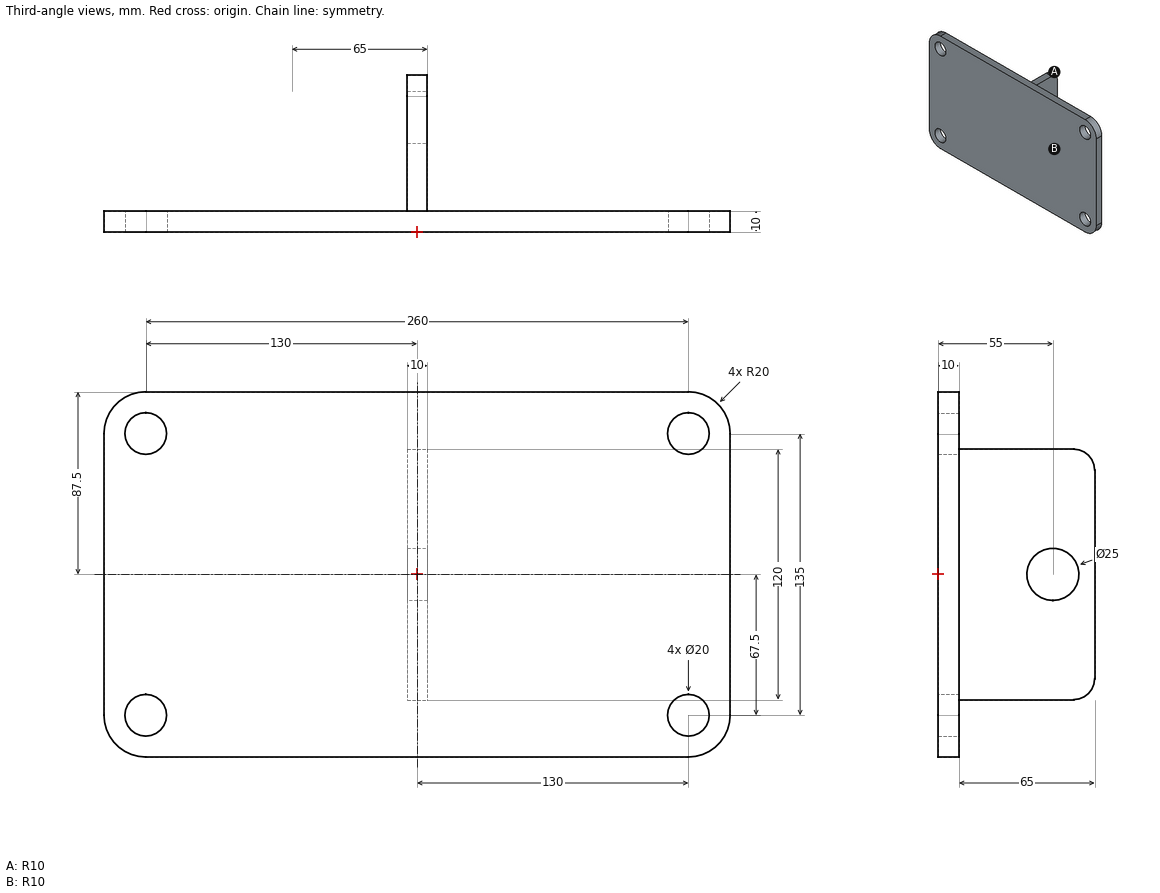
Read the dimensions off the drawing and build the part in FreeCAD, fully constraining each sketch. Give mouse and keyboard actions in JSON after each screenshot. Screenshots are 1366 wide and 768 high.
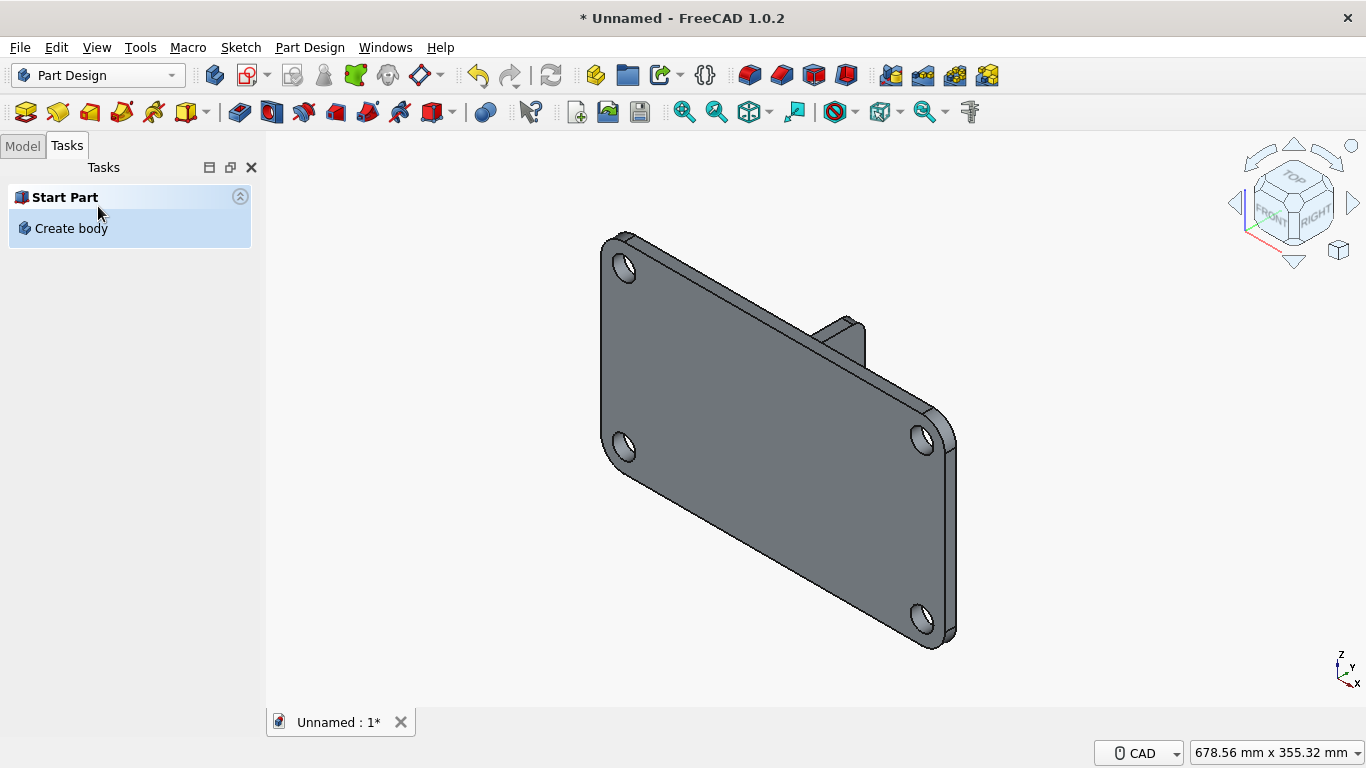
{"action": "key", "text": "3"}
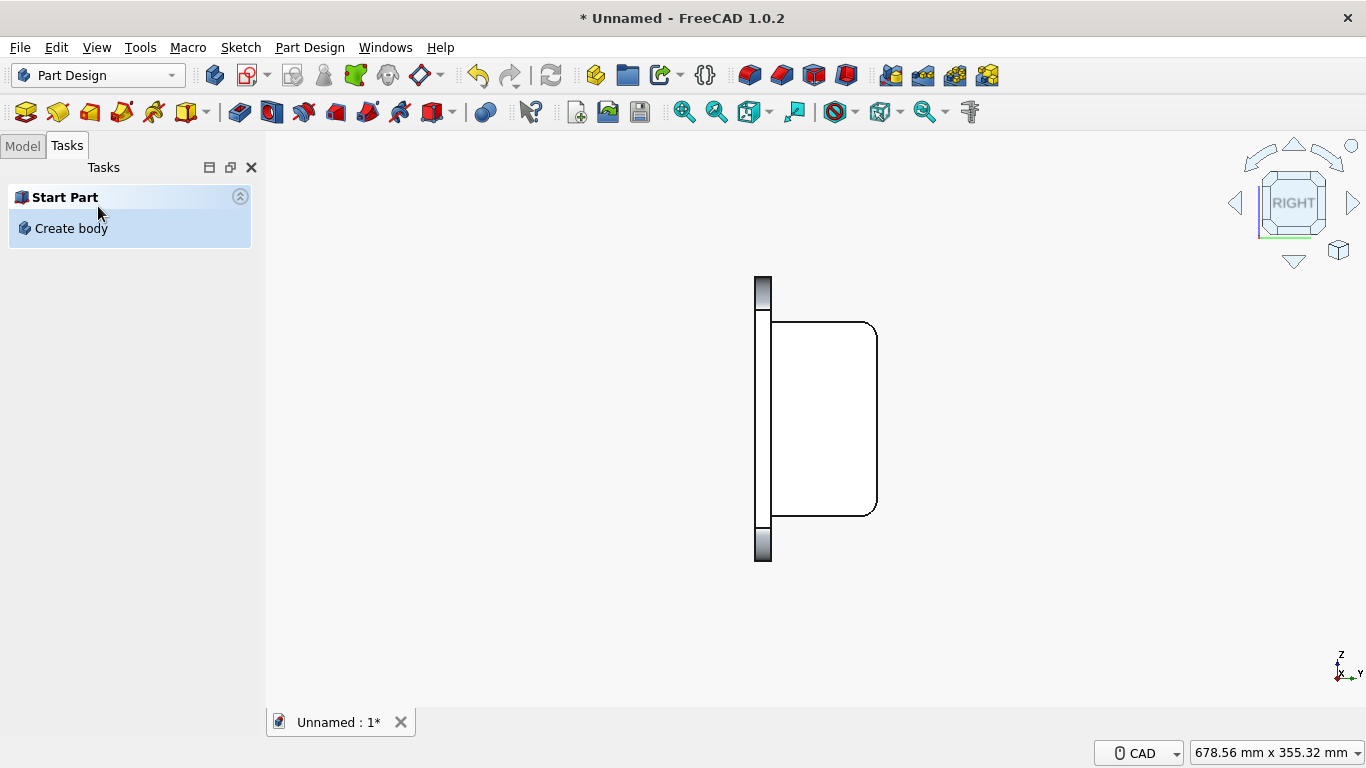
{"action": "left_click", "coordinate": [824, 446]}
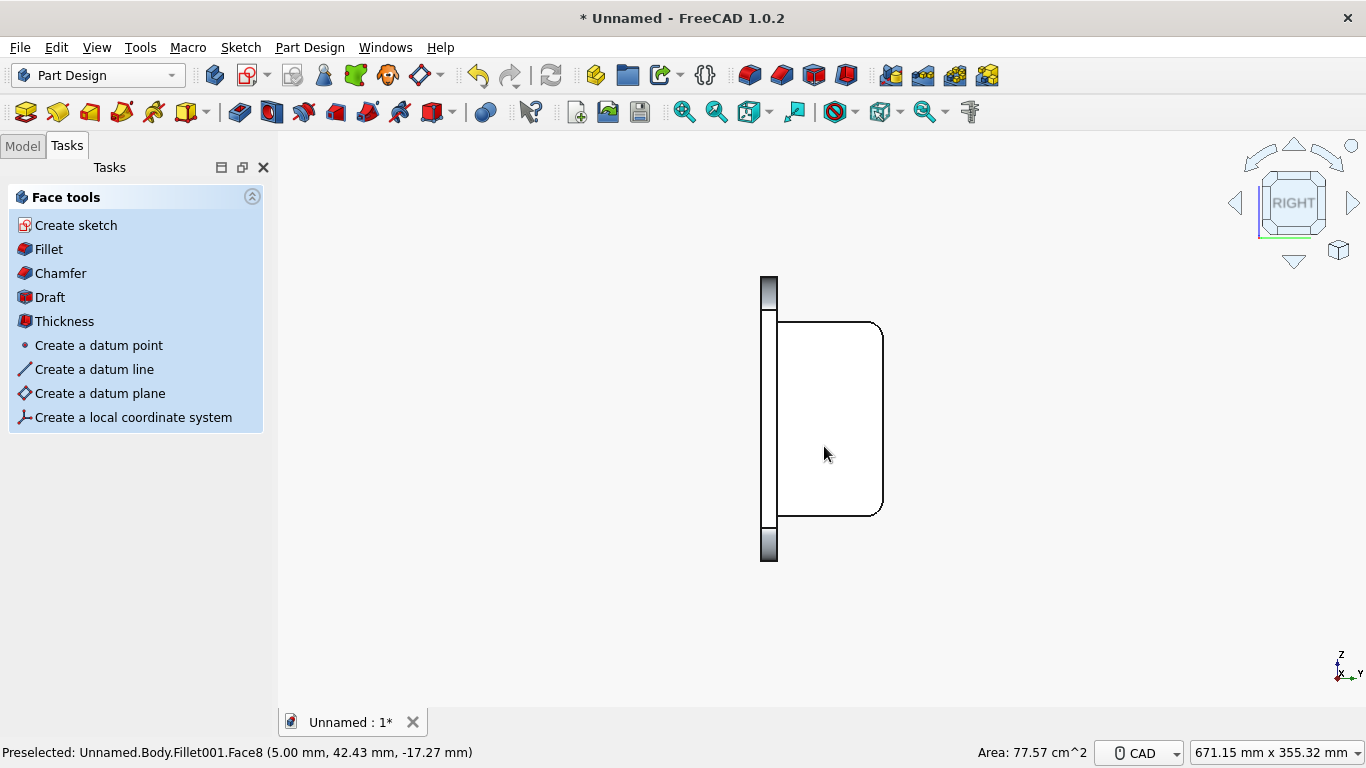
{"action": "left_click", "coordinate": [248, 76]}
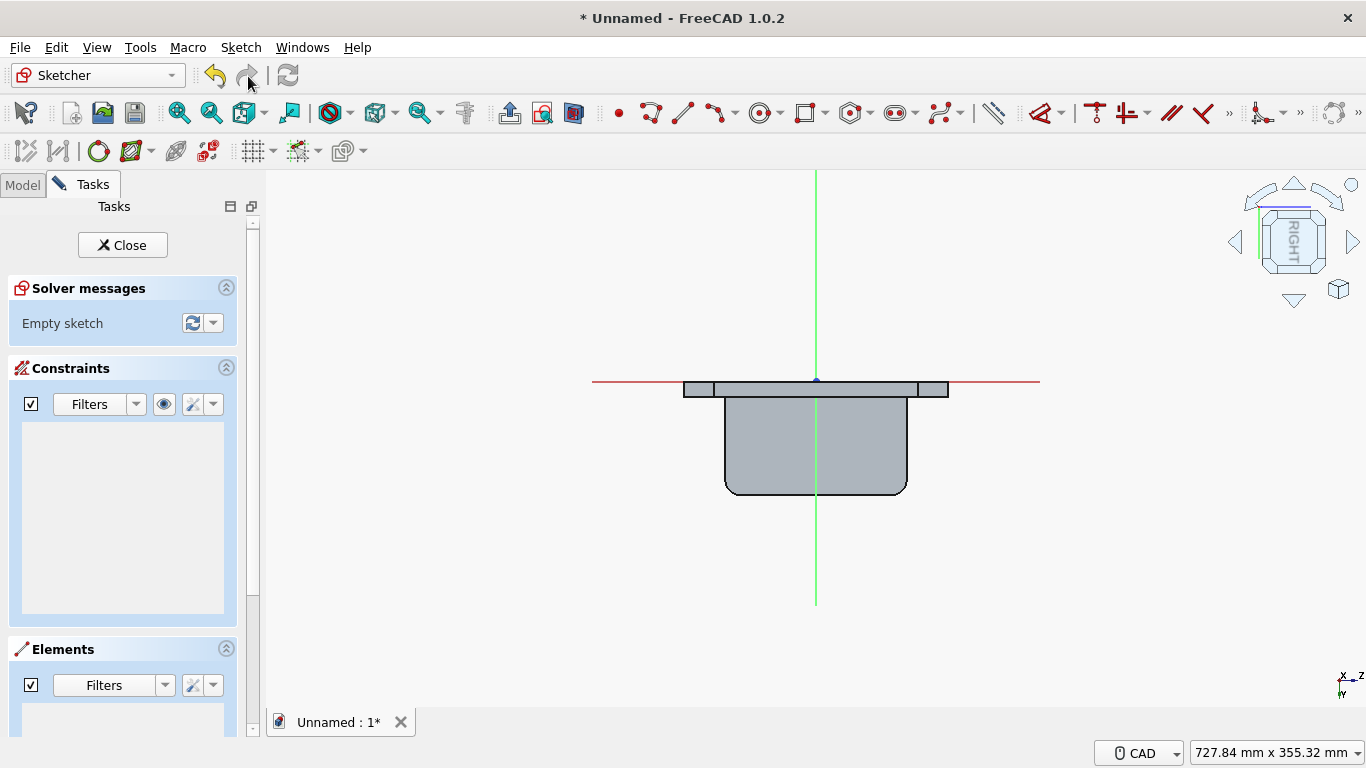
{"action": "scroll", "coordinate": [825, 468], "scroll_direction": "up", "scroll_amount": 11}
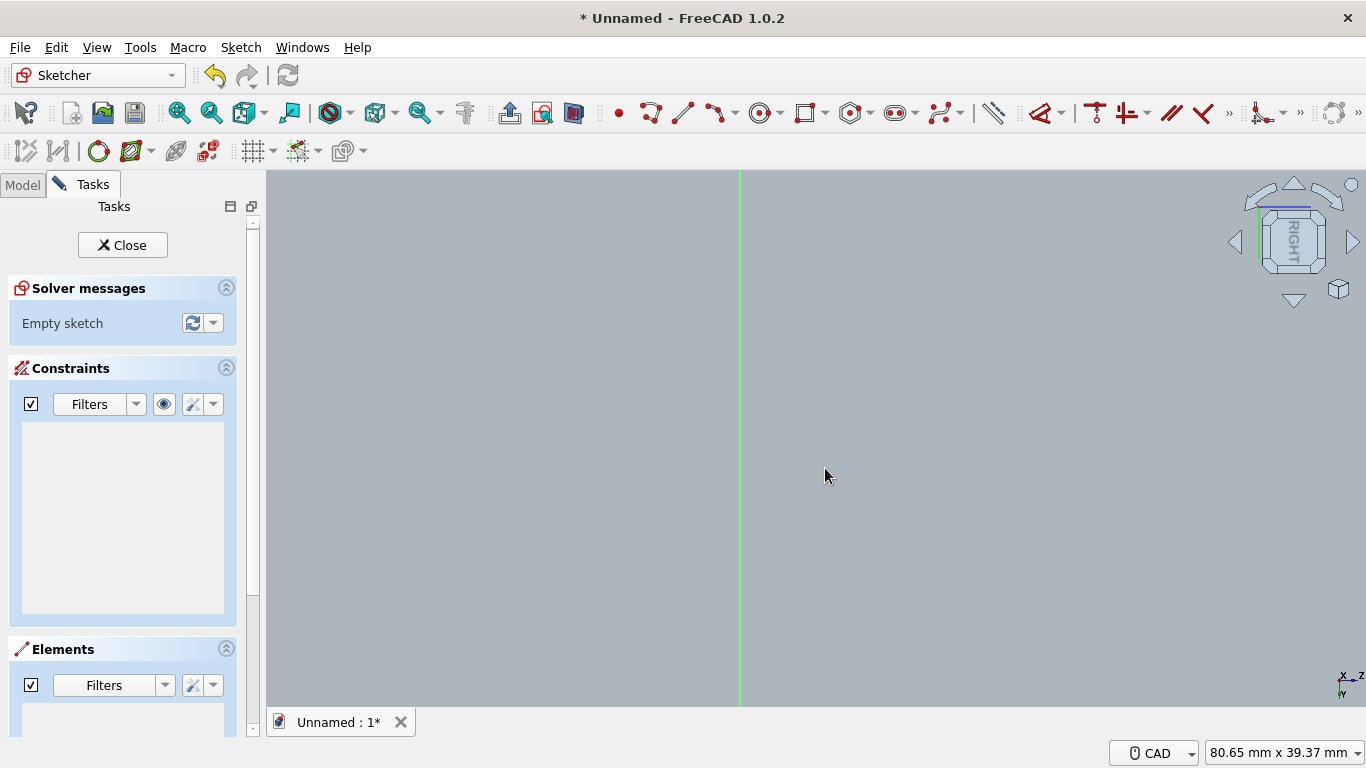
{"action": "left_click", "coordinate": [760, 114]}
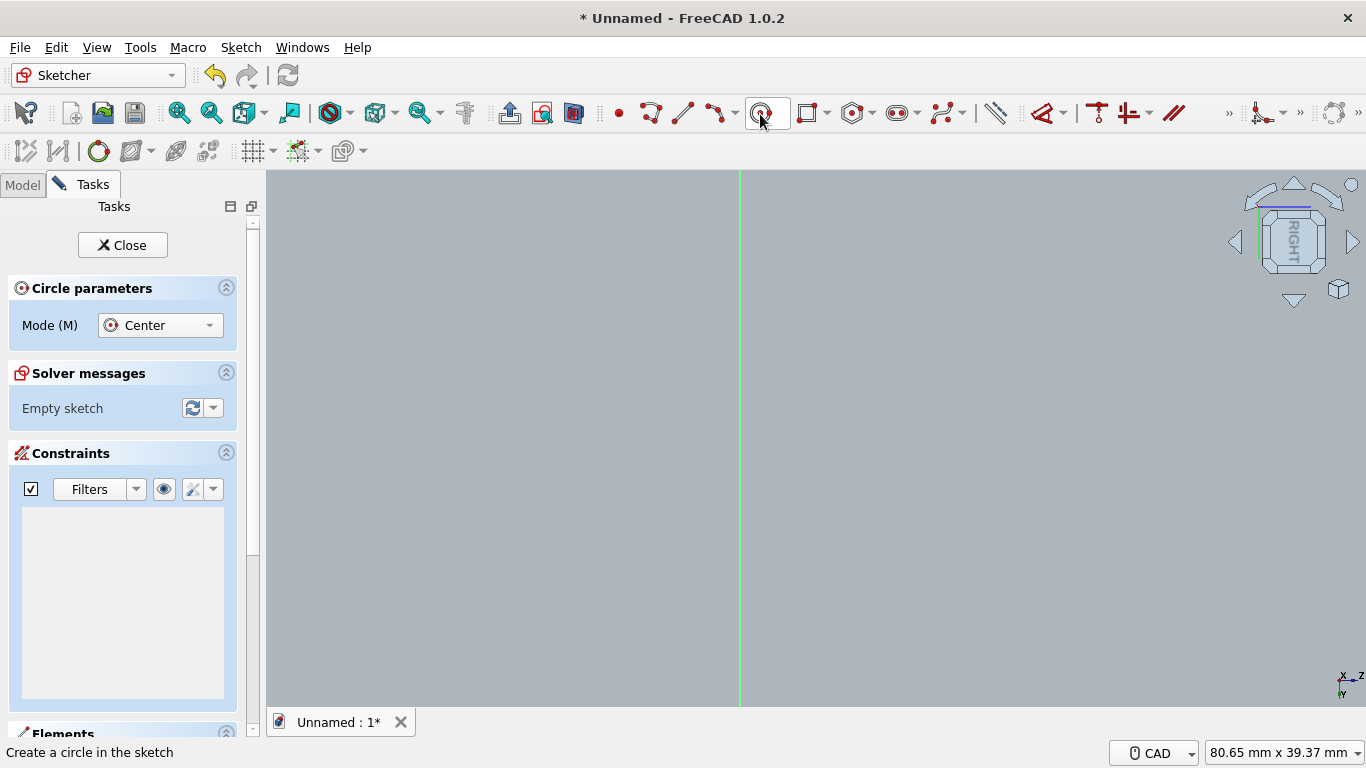
{"action": "left_click", "coordinate": [740, 436]}
{"action": "left_click", "coordinate": [860, 315]}
{"action": "key", "text": "Escape"}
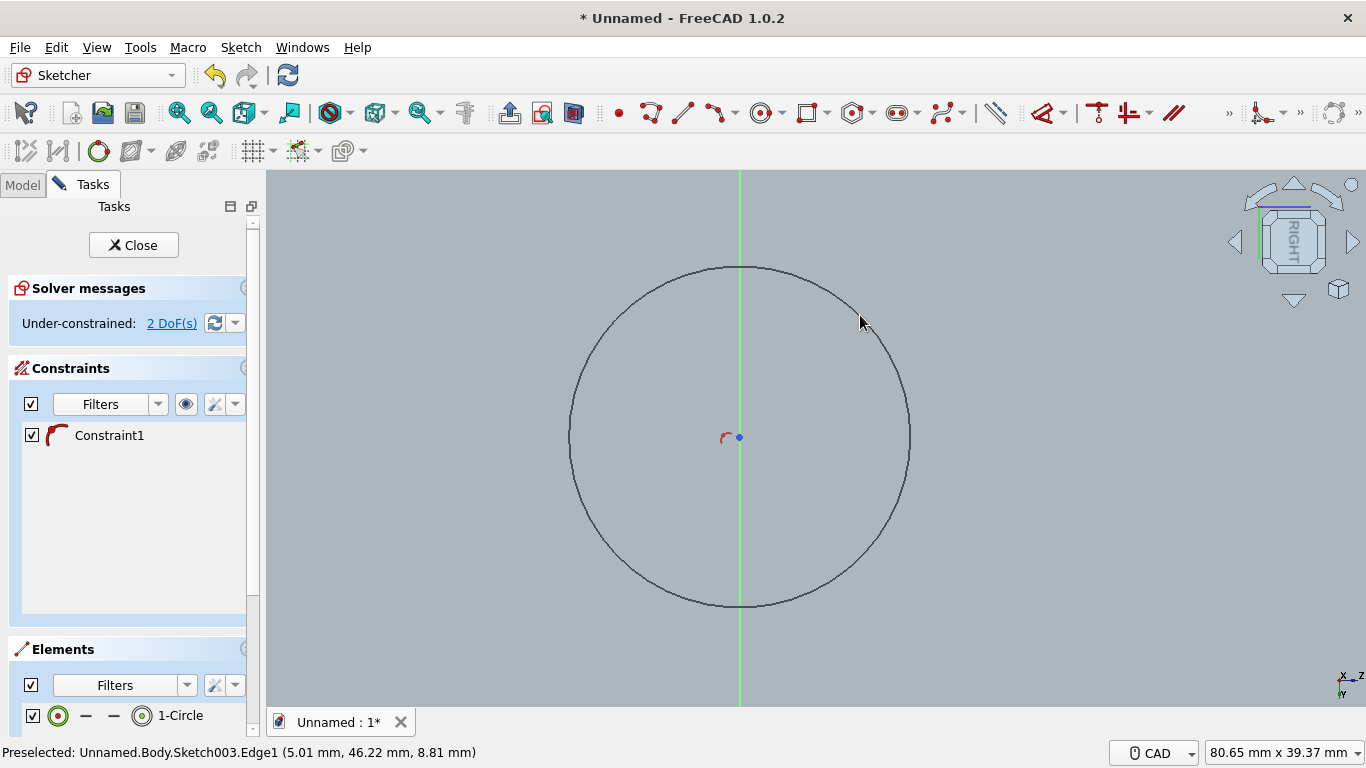
{"action": "left_click", "coordinate": [1042, 114]}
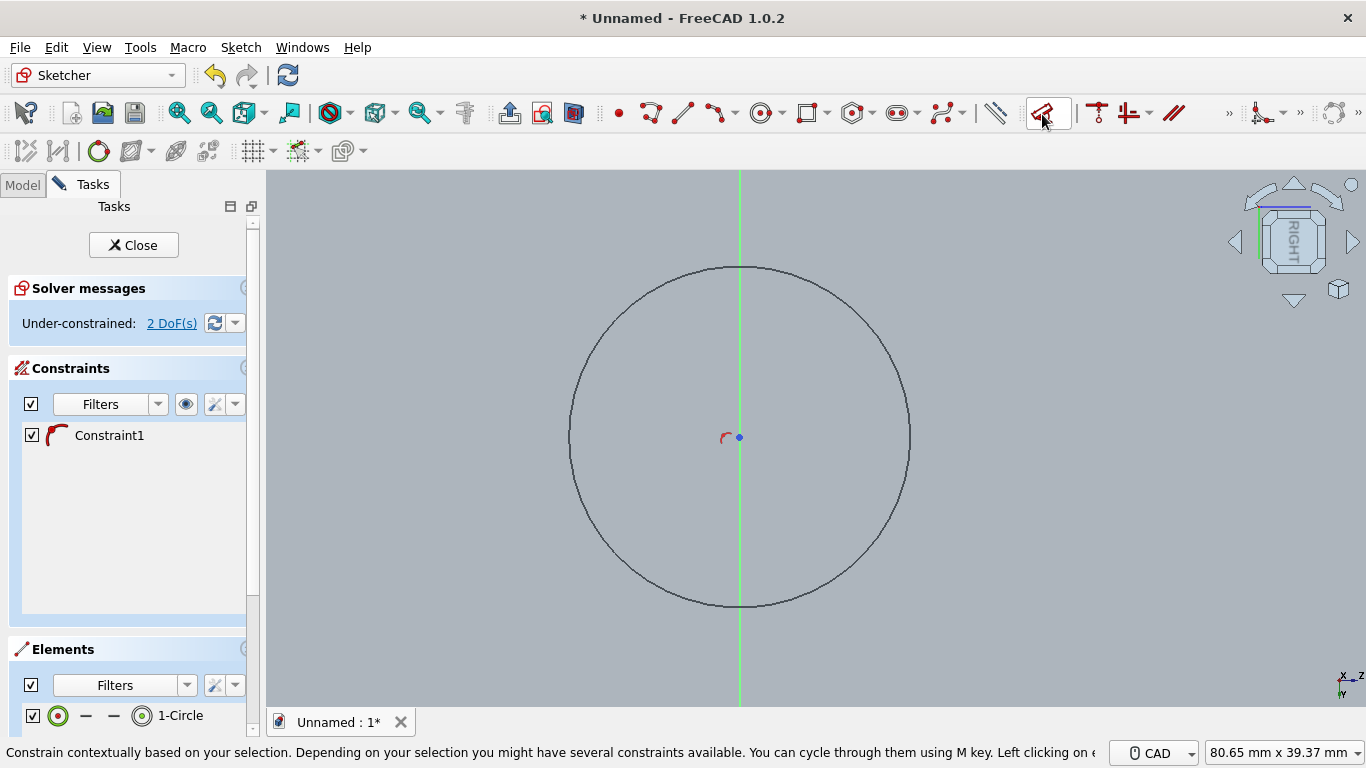
{"action": "left_click", "coordinate": [860, 316]}
{"action": "left_click", "coordinate": [883, 293]}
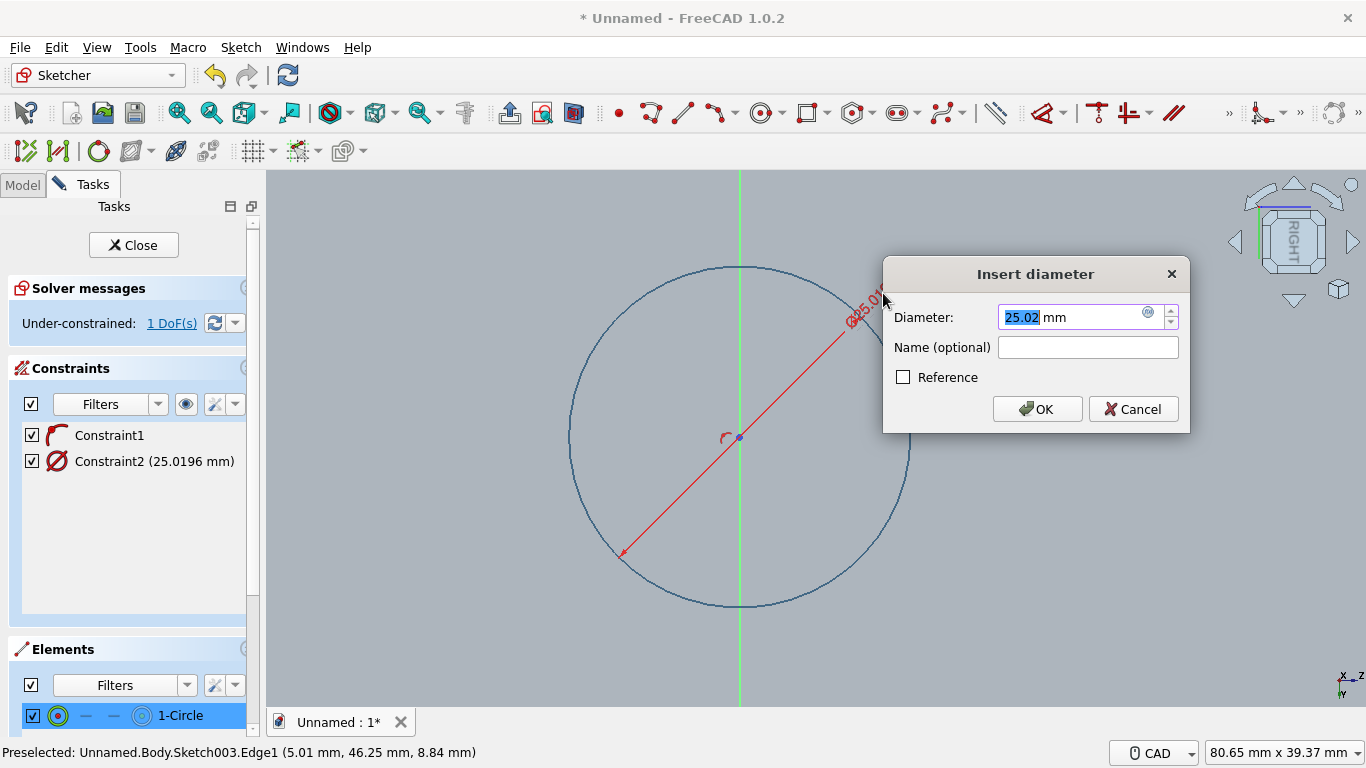
{"action": "type", "text": "25"}
{"action": "key", "text": "Return"}